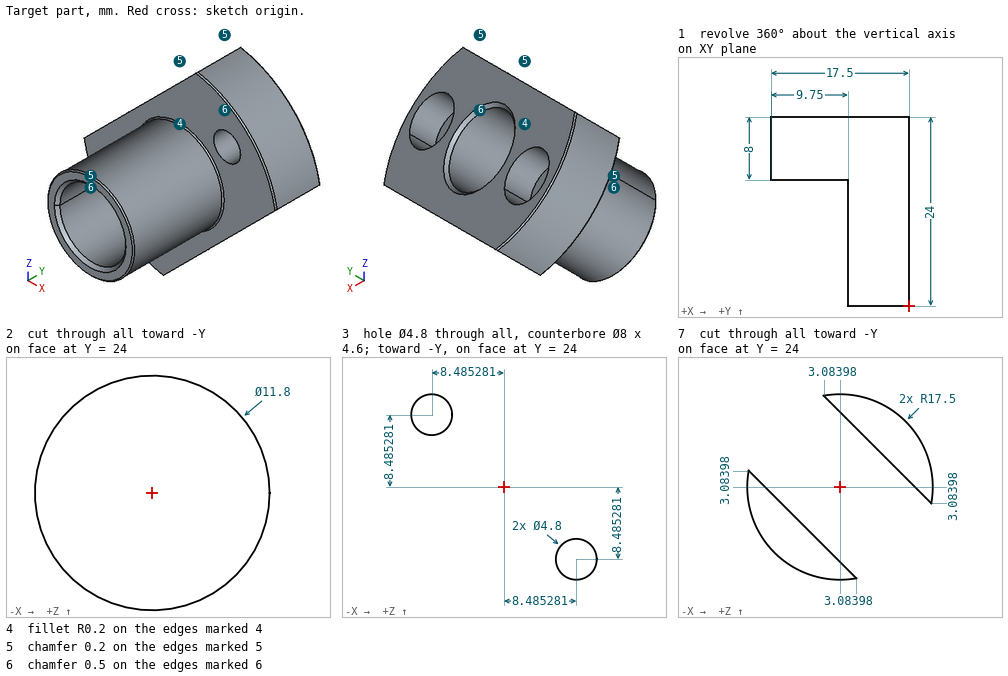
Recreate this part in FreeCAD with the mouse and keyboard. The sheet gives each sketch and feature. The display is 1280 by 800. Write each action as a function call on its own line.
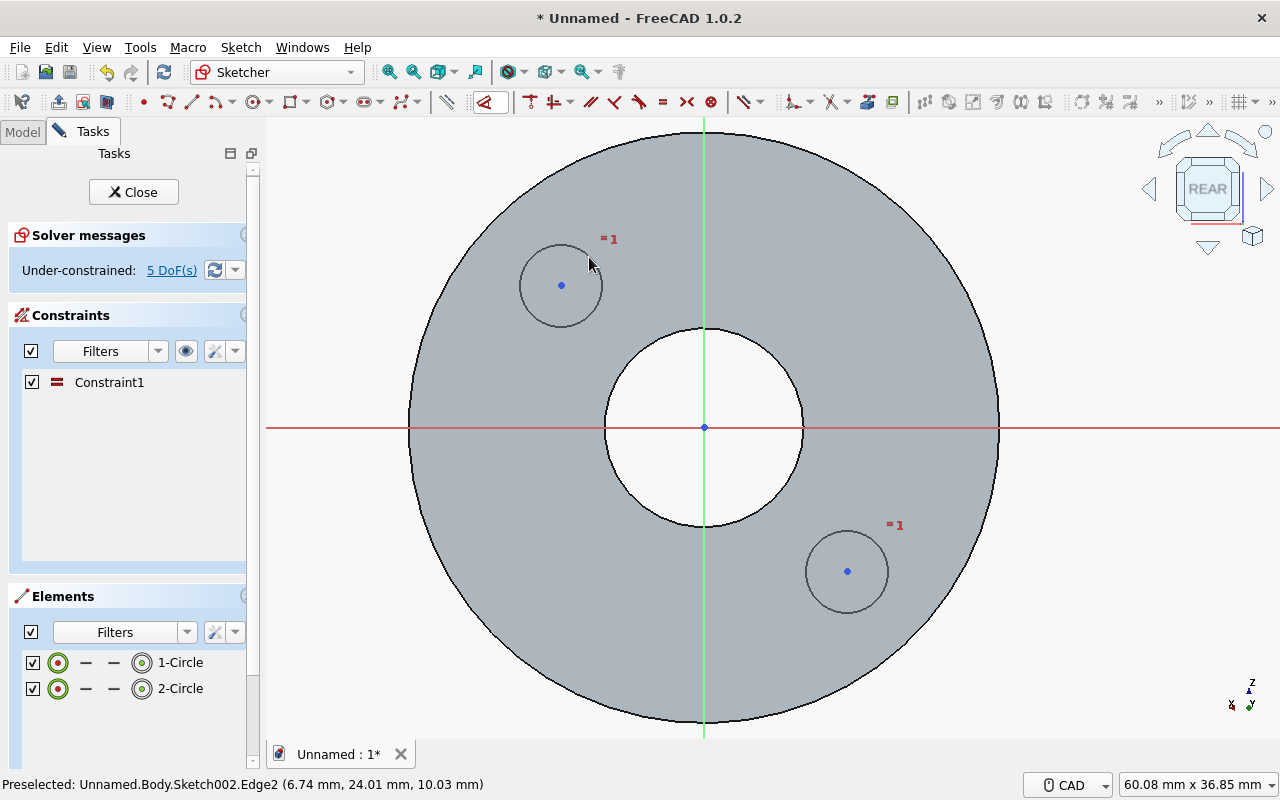
click(876, 543)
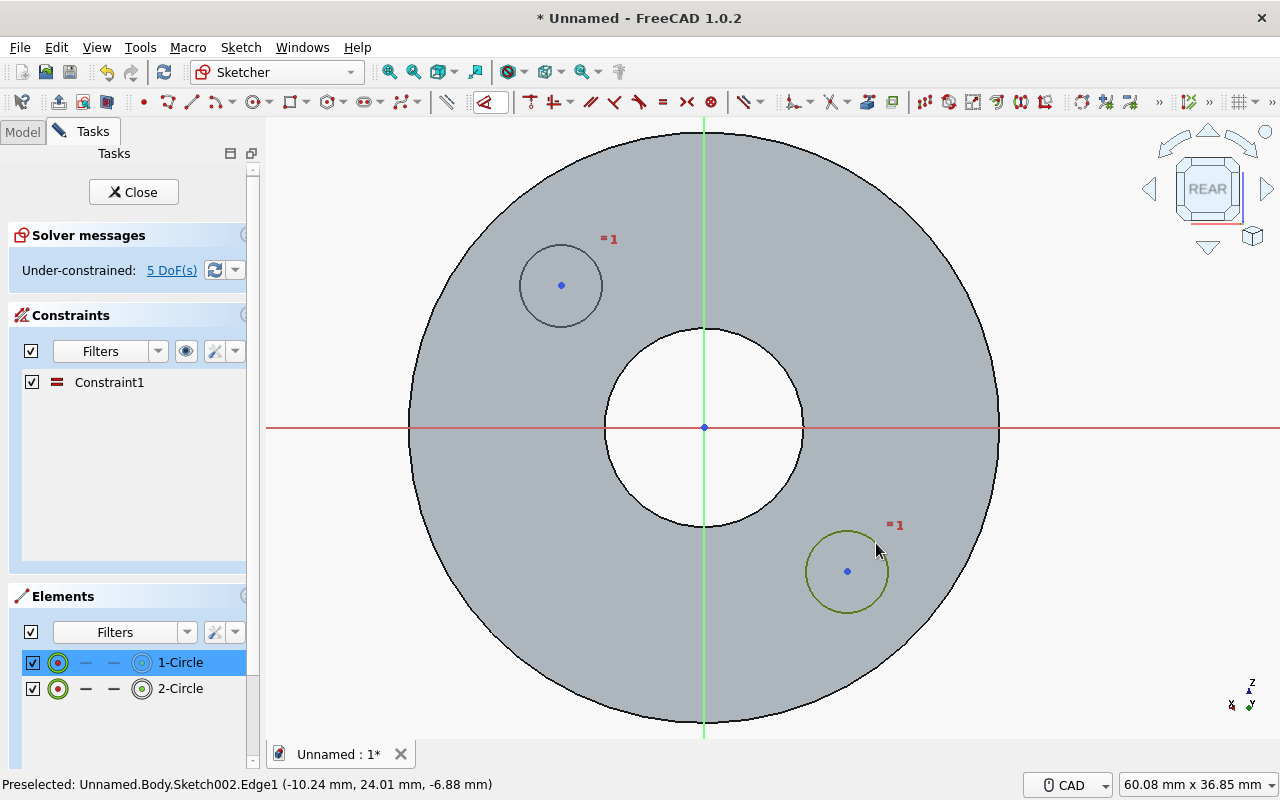
key(k)
key(o)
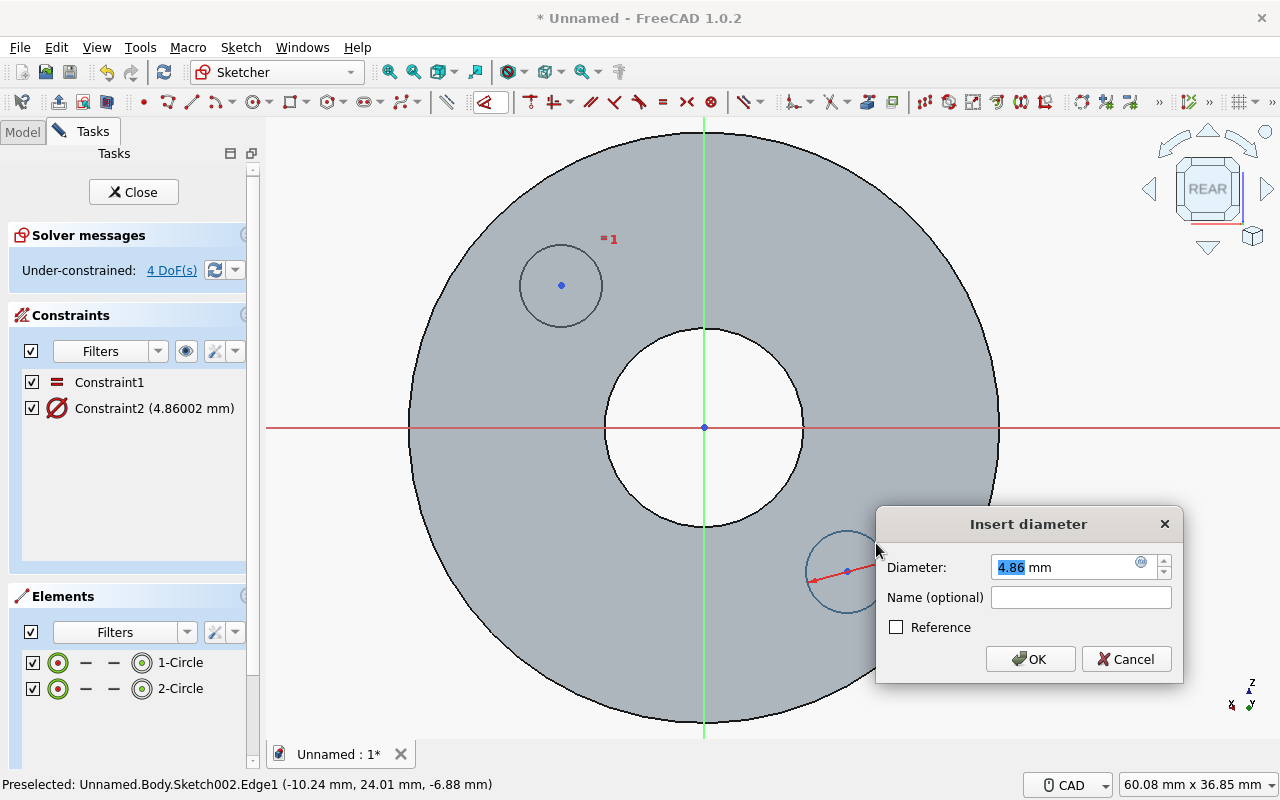
text(4.8)
key(Return)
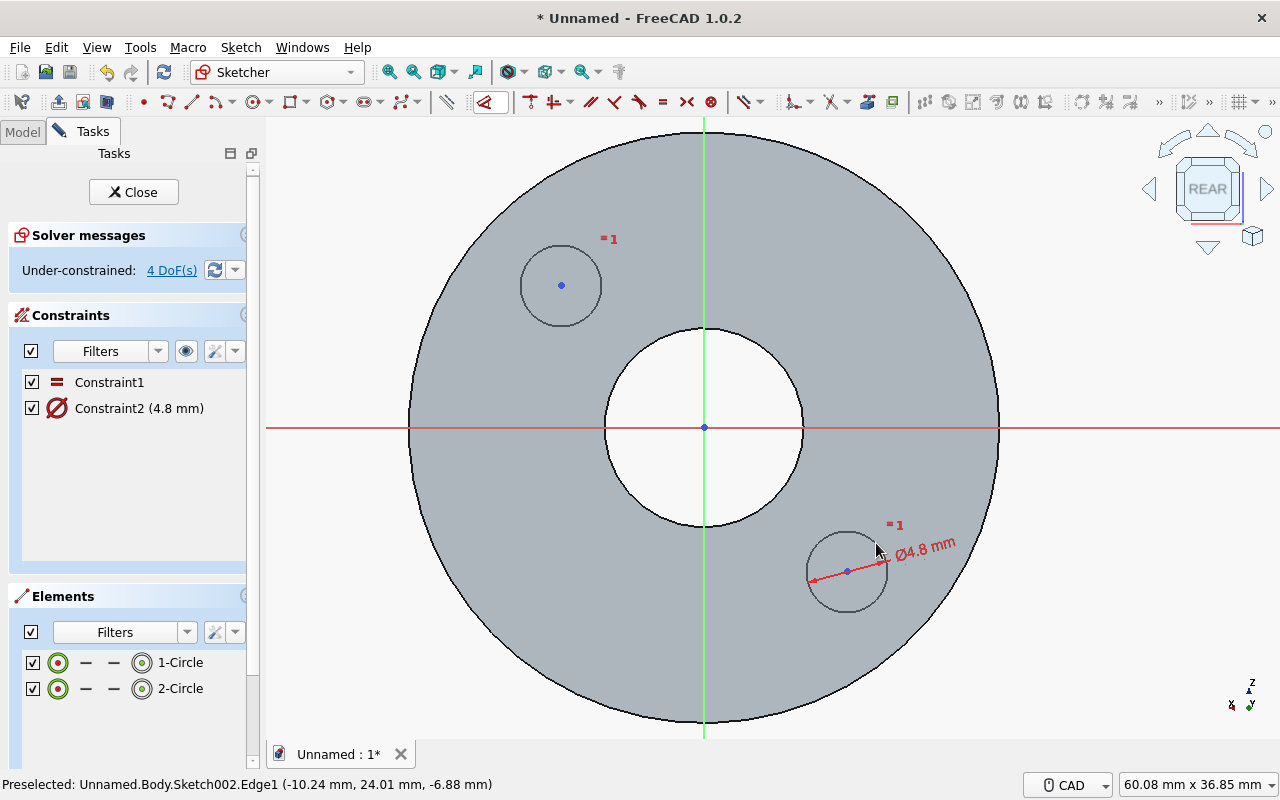
click(847, 572)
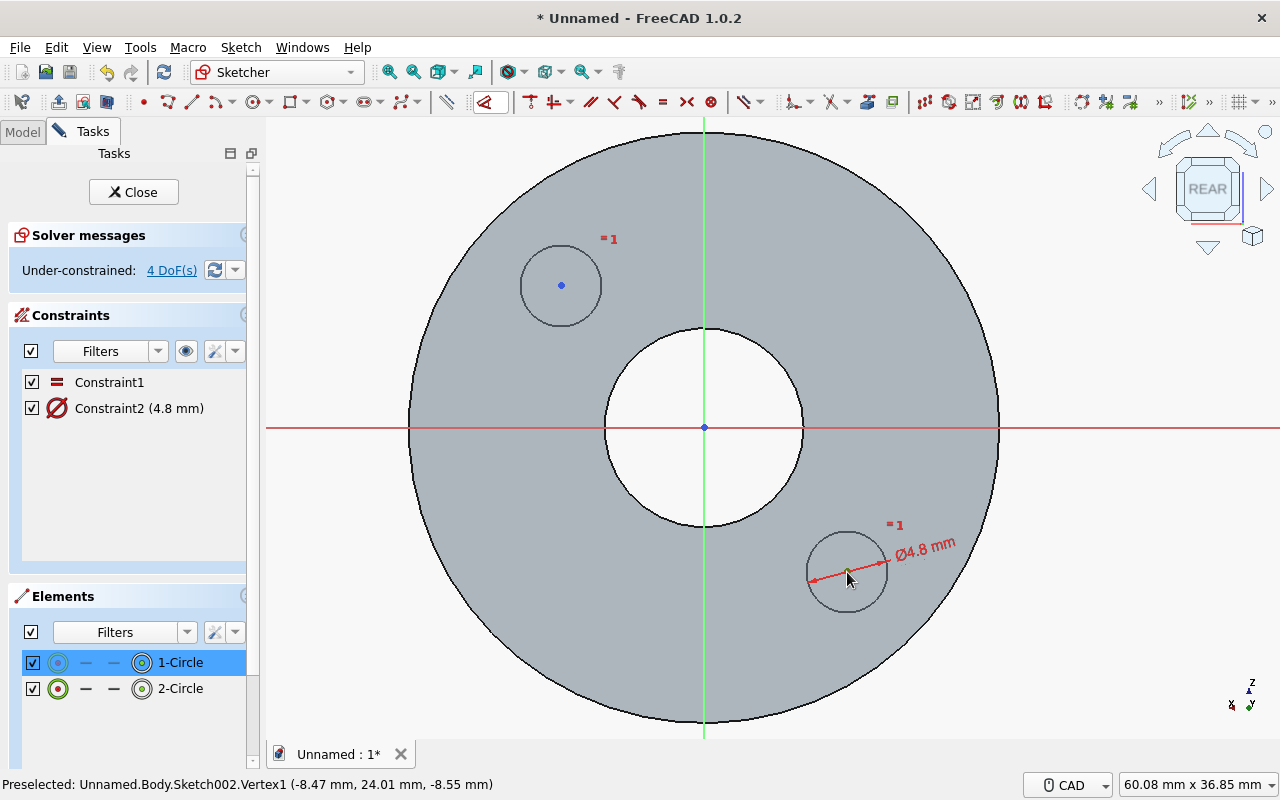
key(l)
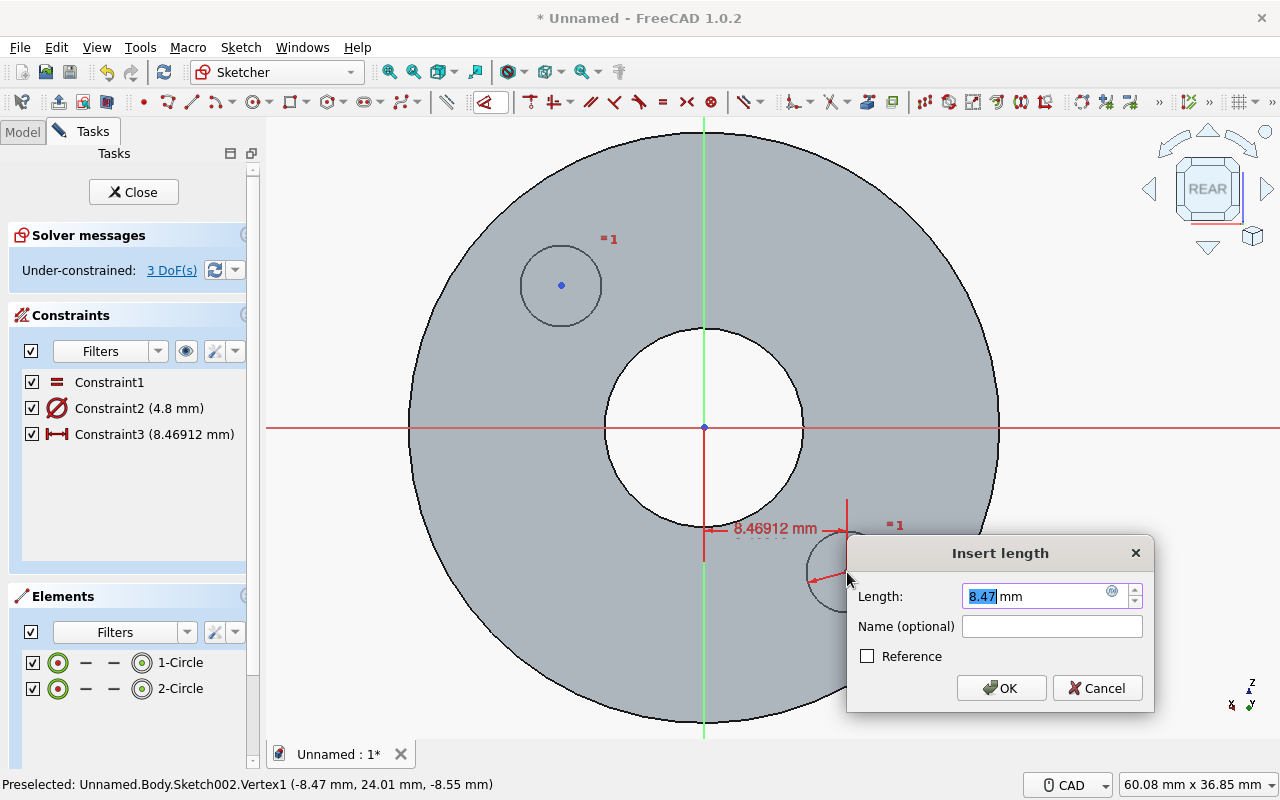
text(8.485281)
key(Return)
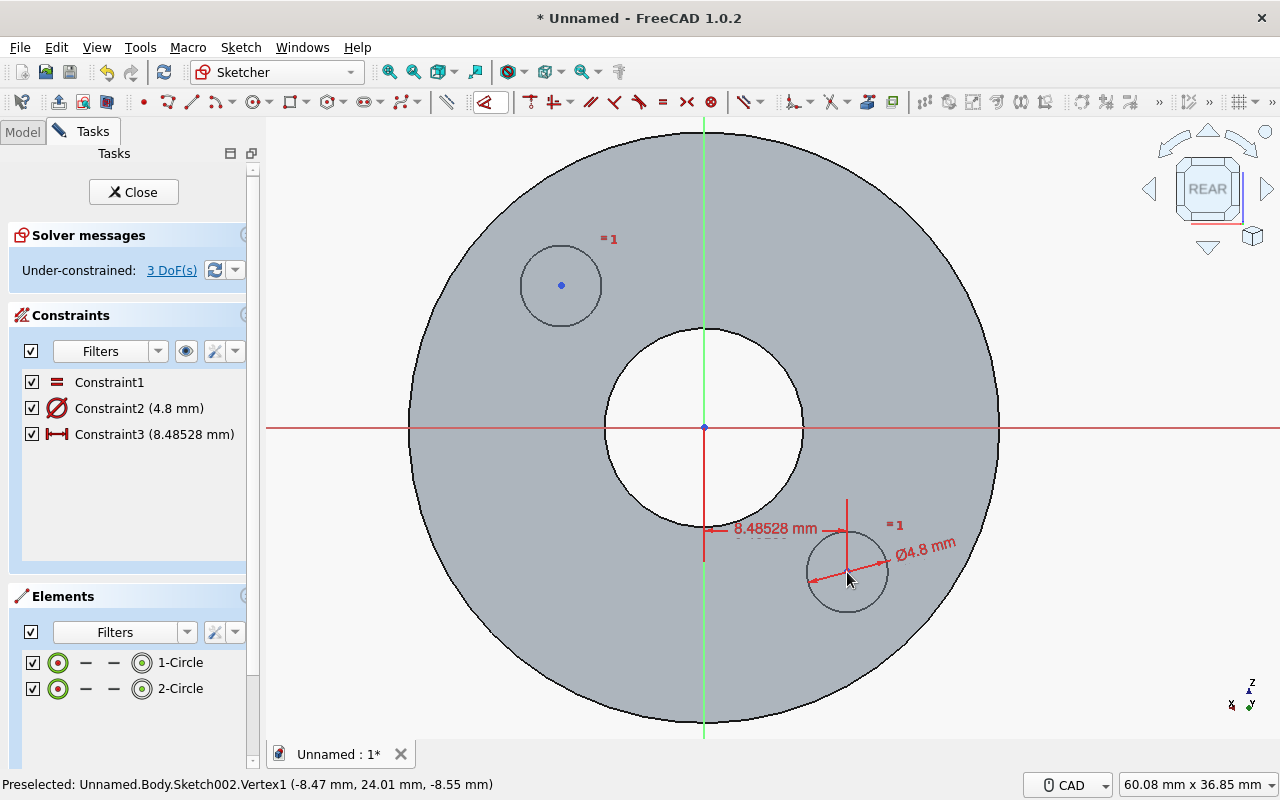
click(847, 572)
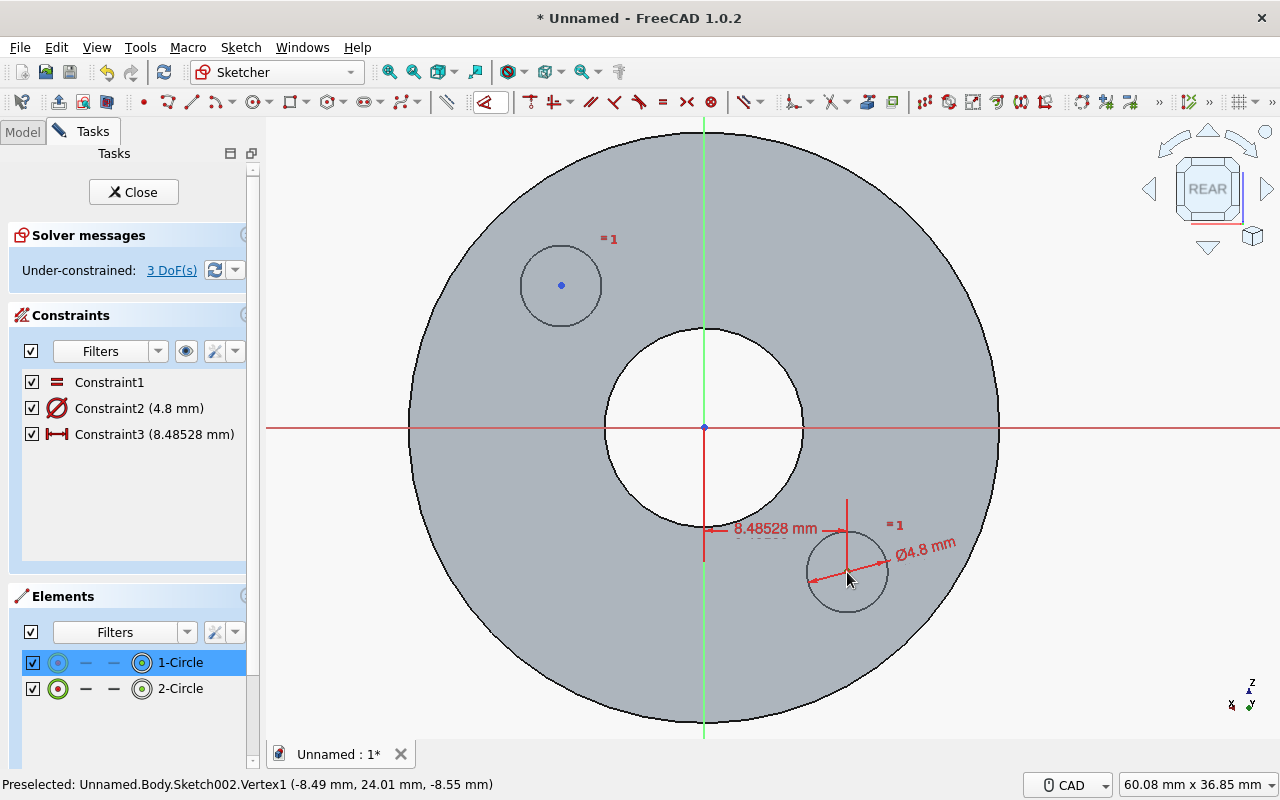
key(i)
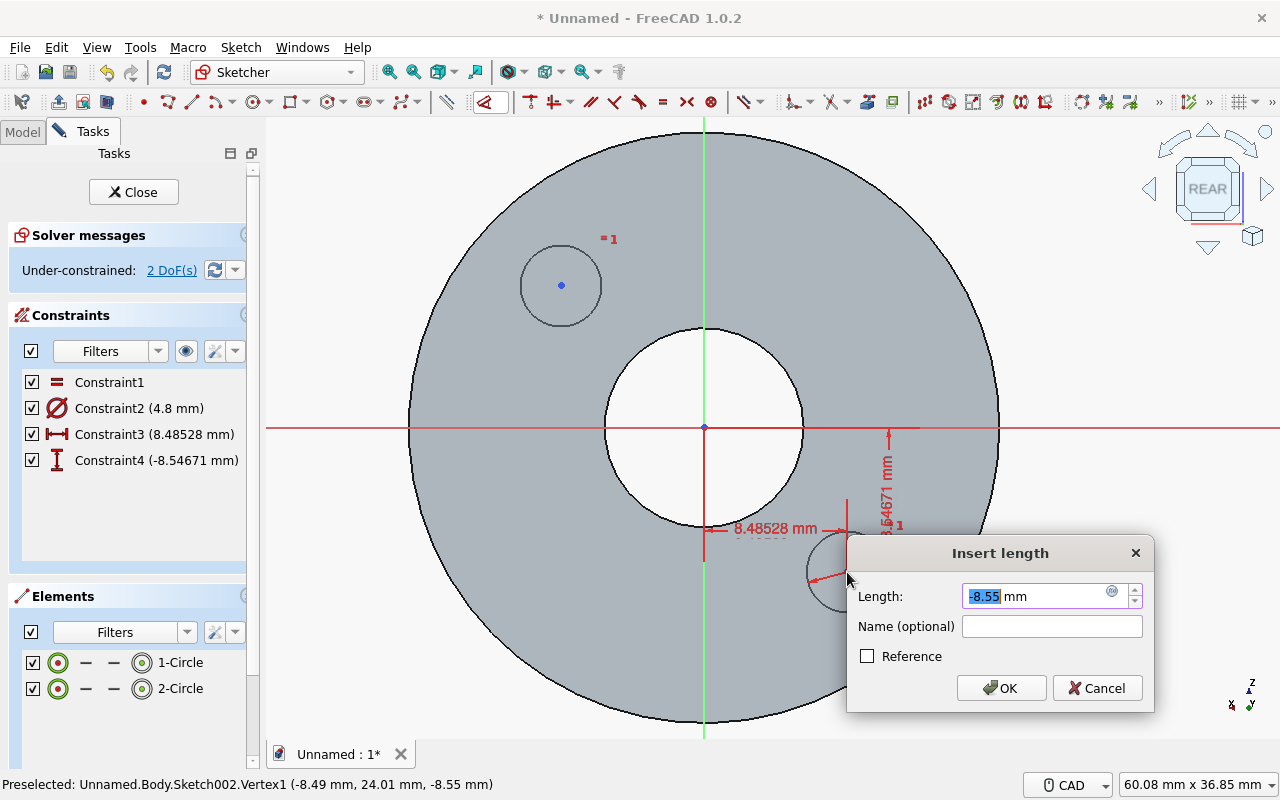
text(-8.485281)
key(Return)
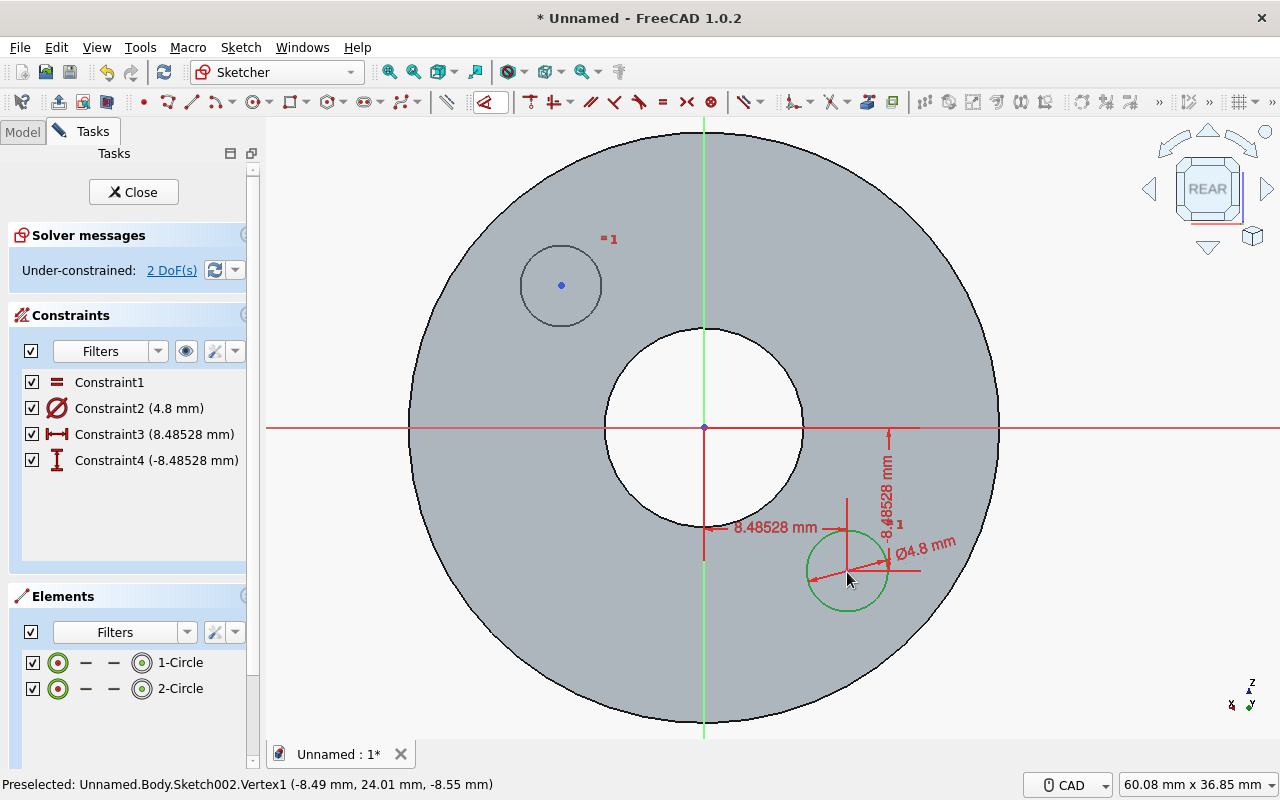
click(561, 286)